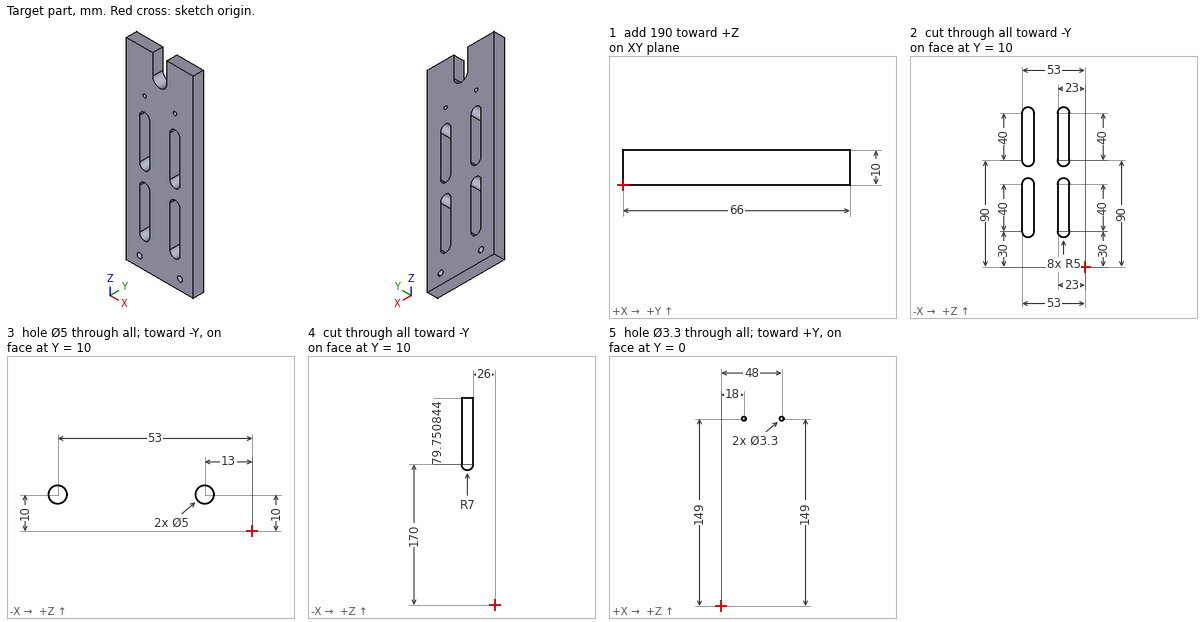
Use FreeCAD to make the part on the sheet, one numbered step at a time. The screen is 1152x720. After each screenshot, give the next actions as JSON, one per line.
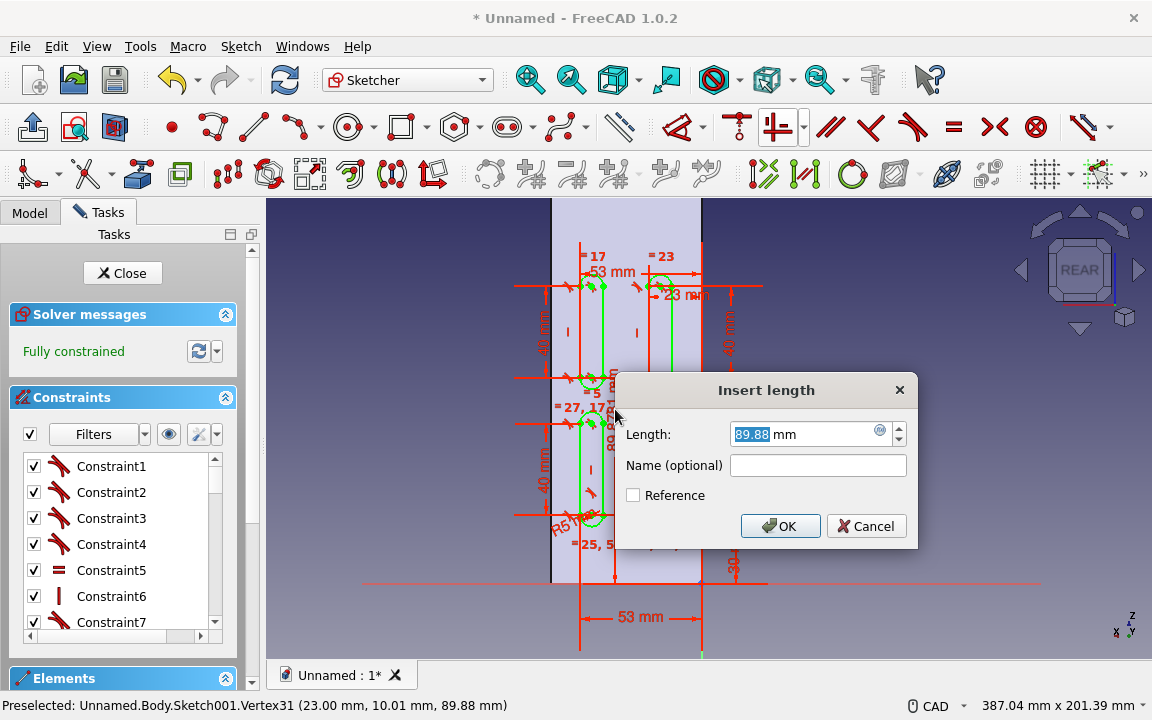
{"action": "type", "text": "90"}
{"action": "key", "text": "Return"}
{"action": "key", "text": "Escape"}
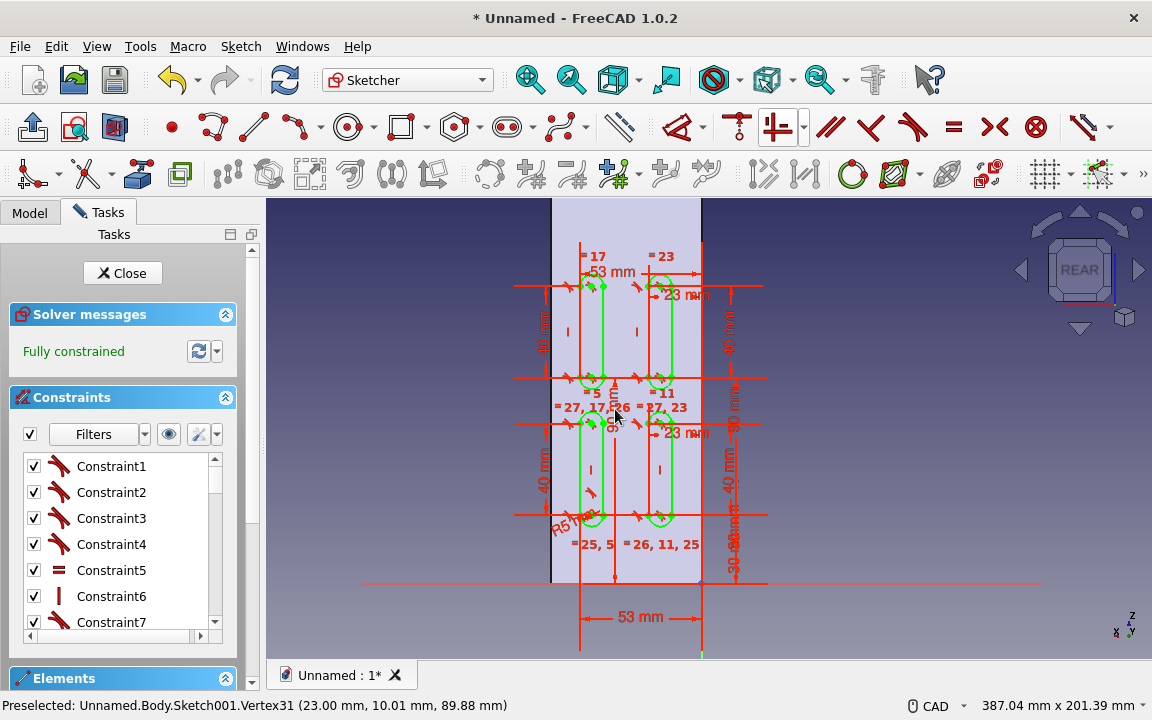
{"action": "left_click", "coordinate": [123, 273]}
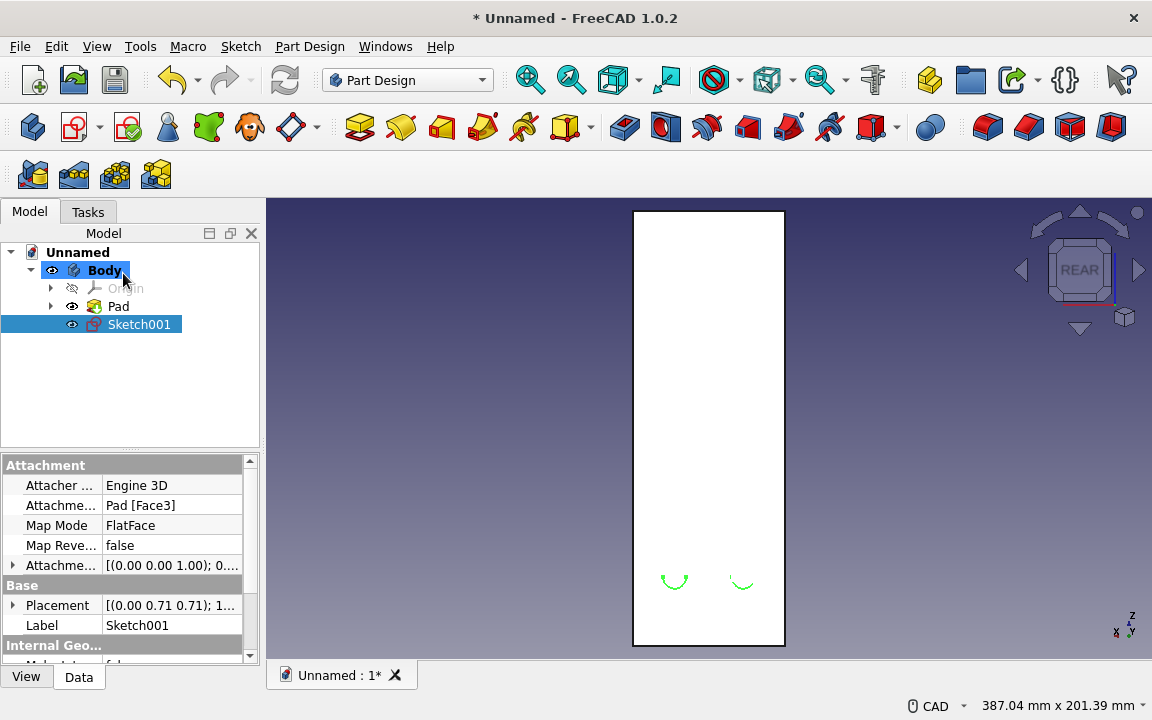
{"action": "left_click", "coordinate": [625, 128]}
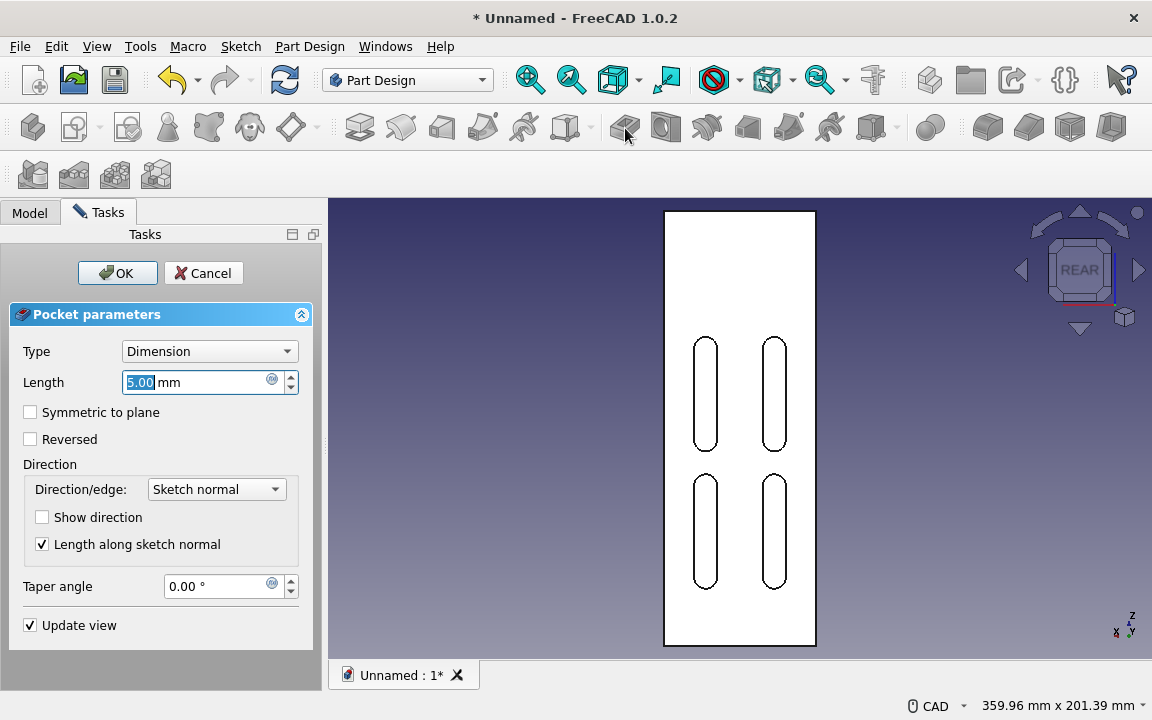
{"action": "left_click", "coordinate": [210, 352]}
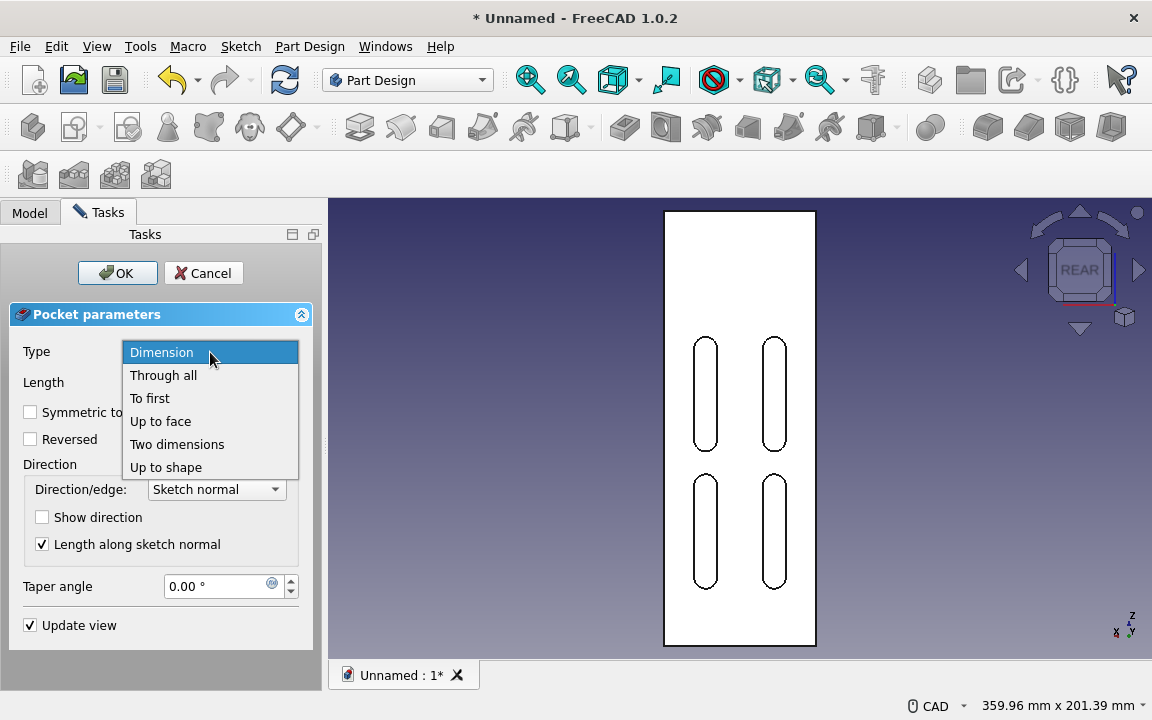
{"action": "left_click", "coordinate": [208, 376]}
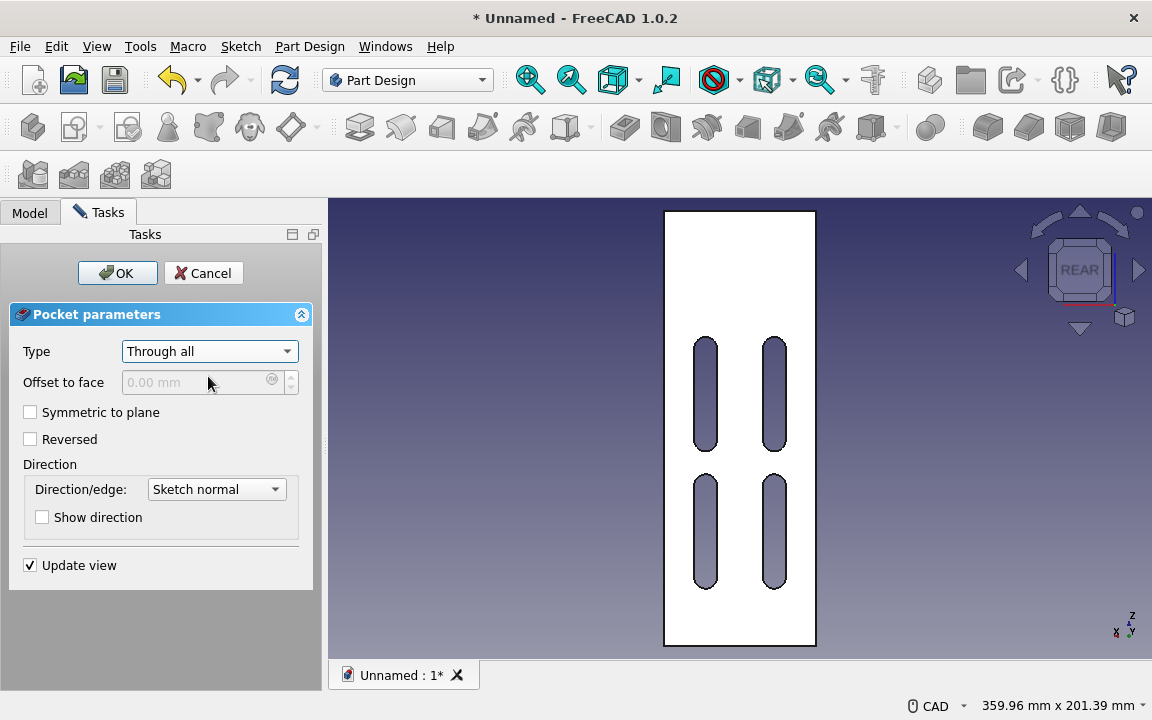
{"action": "left_click", "coordinate": [118, 273]}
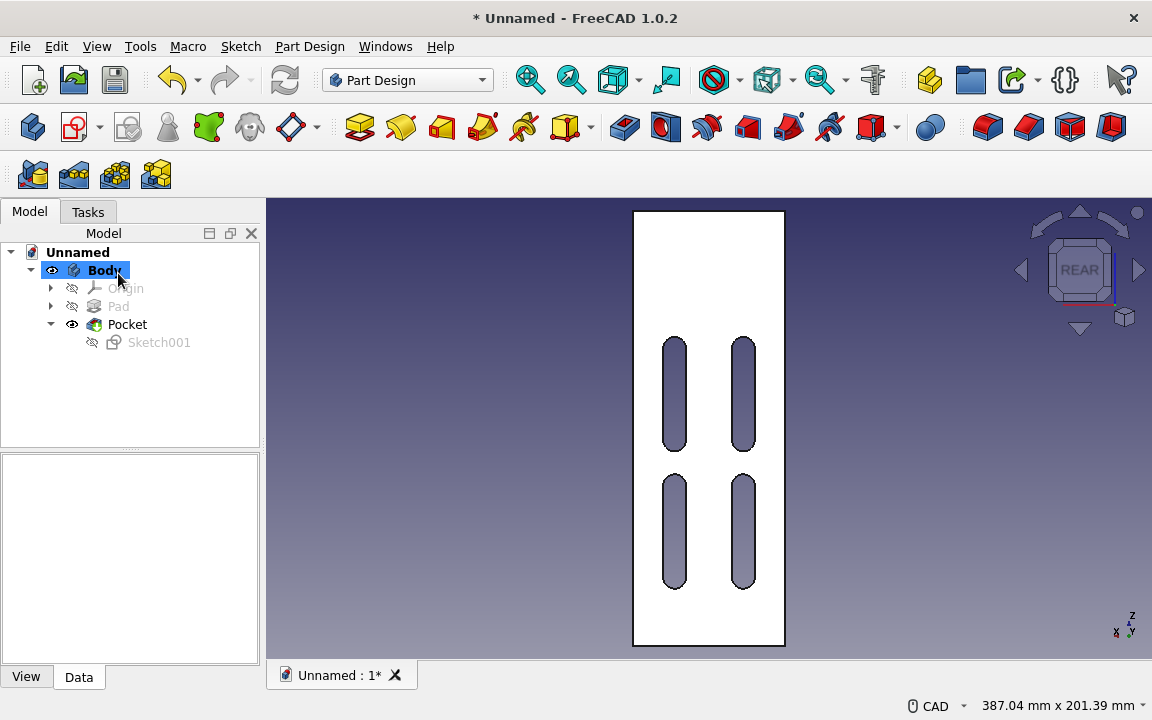
{"action": "left_click", "coordinate": [709, 303]}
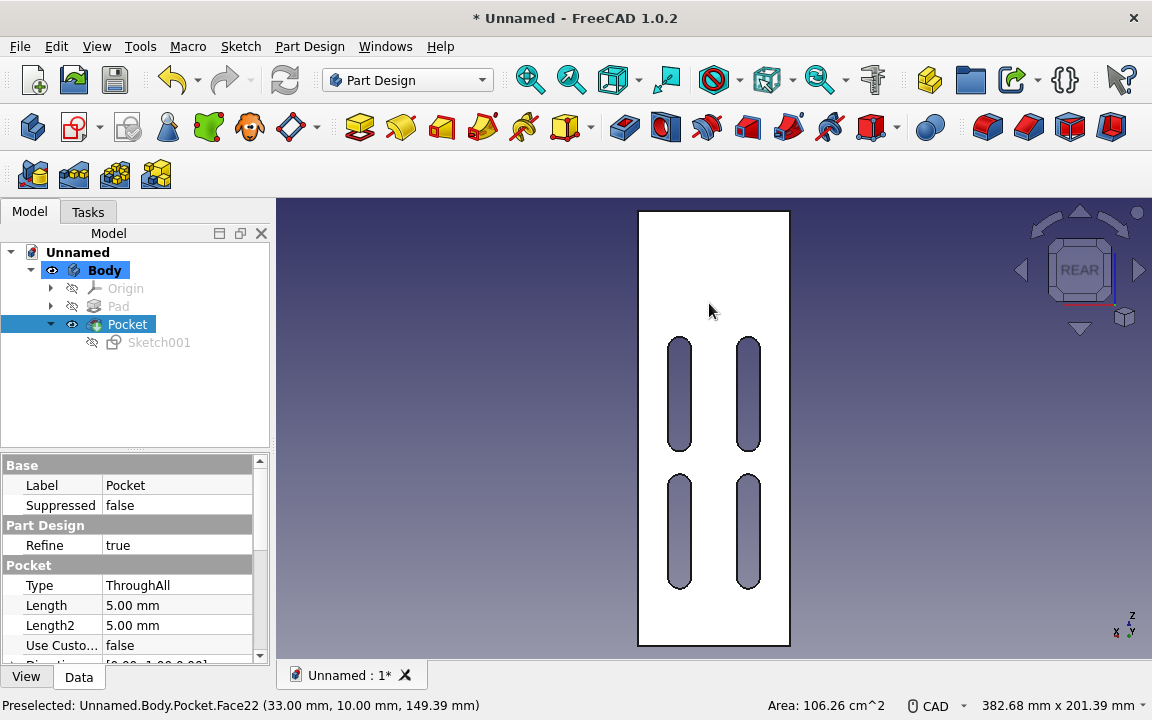
{"action": "left_click", "coordinate": [74, 128]}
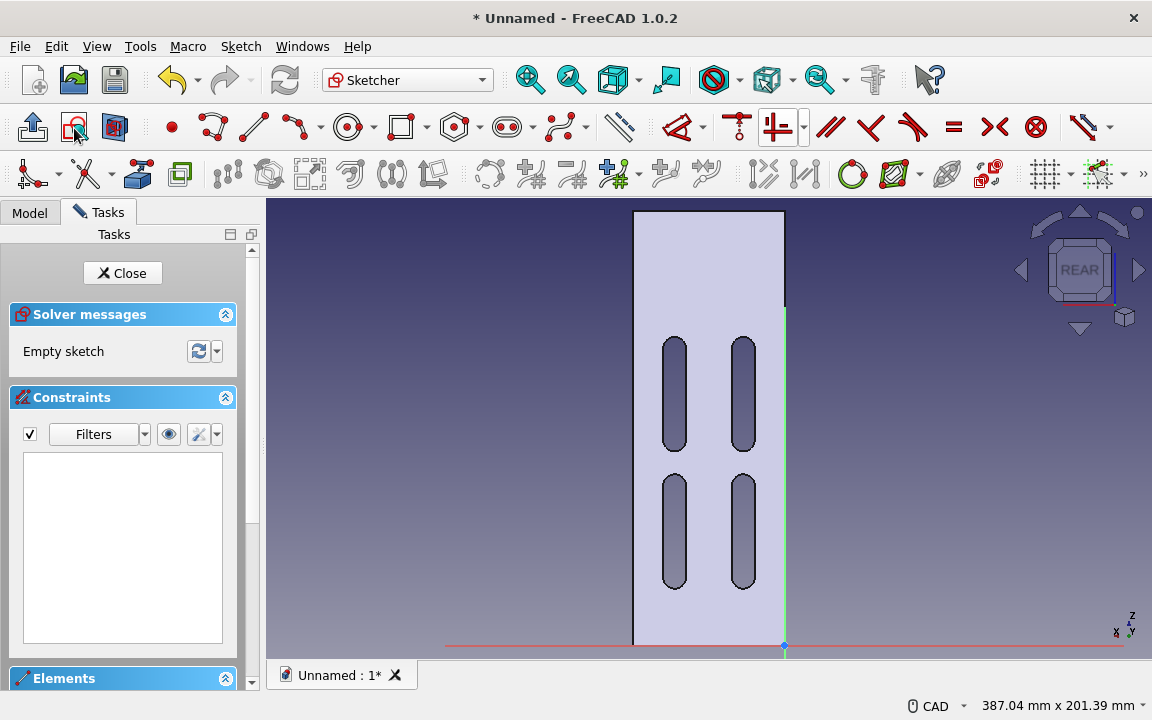
{"action": "scroll", "coordinate": [640, 428], "scroll_direction": "down", "scroll_amount": 5}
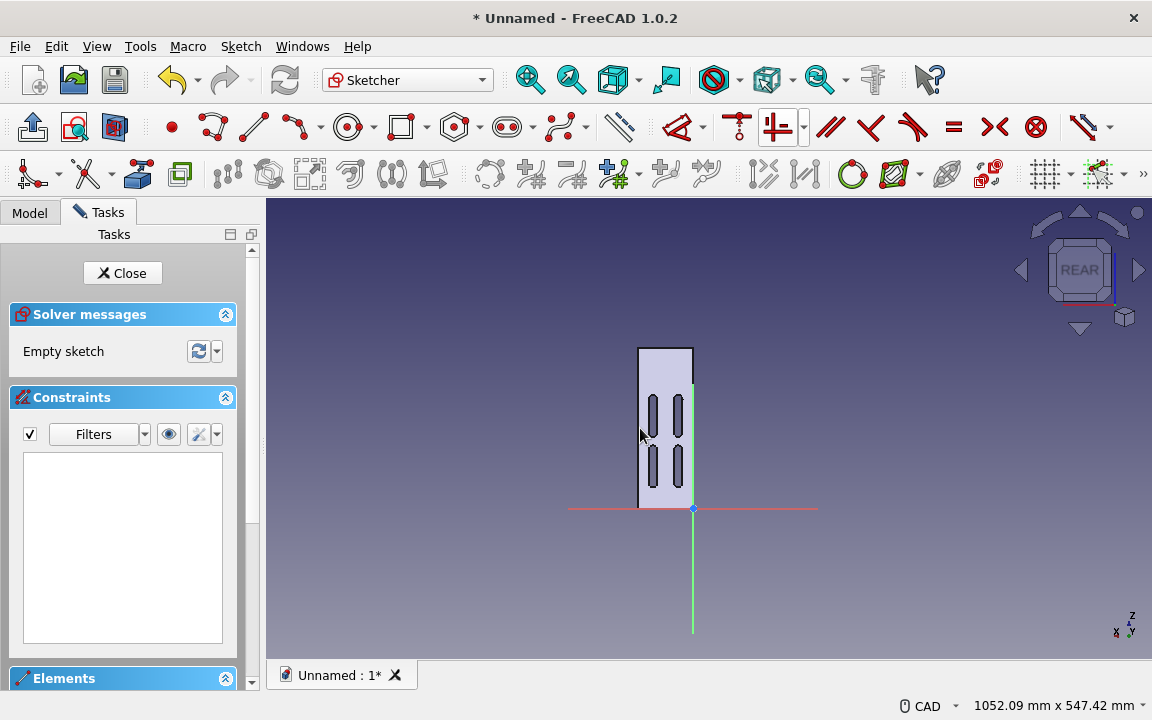
{"action": "scroll", "coordinate": [673, 511], "scroll_direction": "up", "scroll_amount": 12}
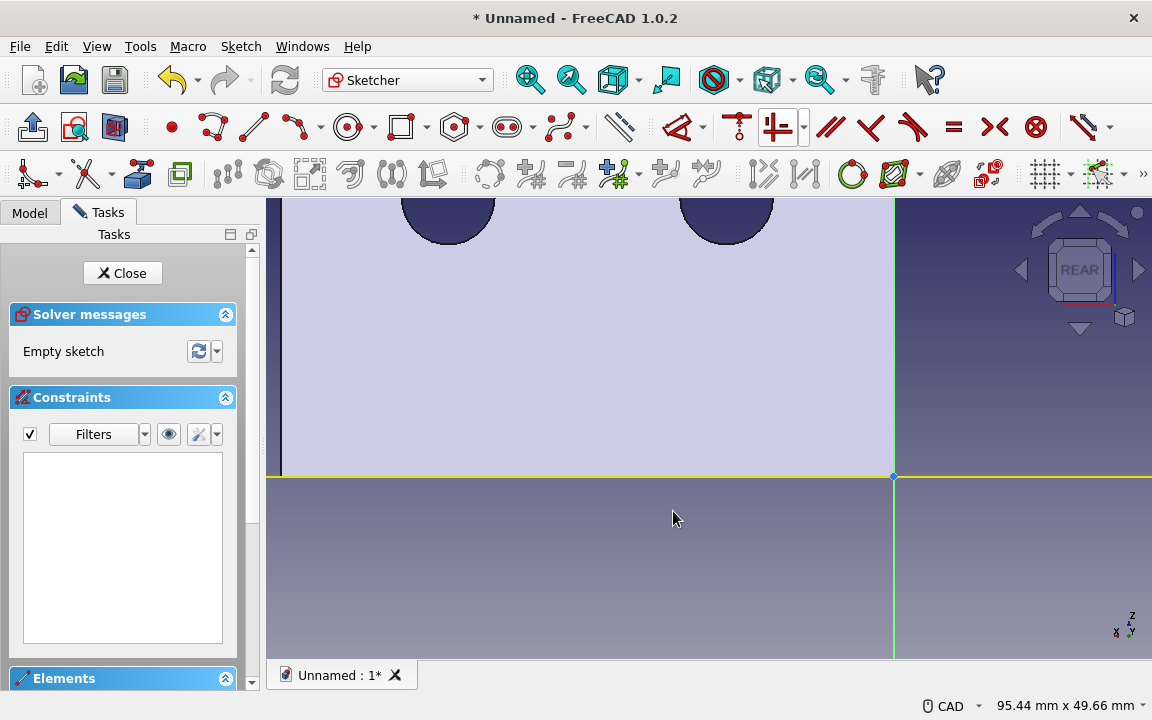
{"action": "left_click", "coordinate": [348, 128]}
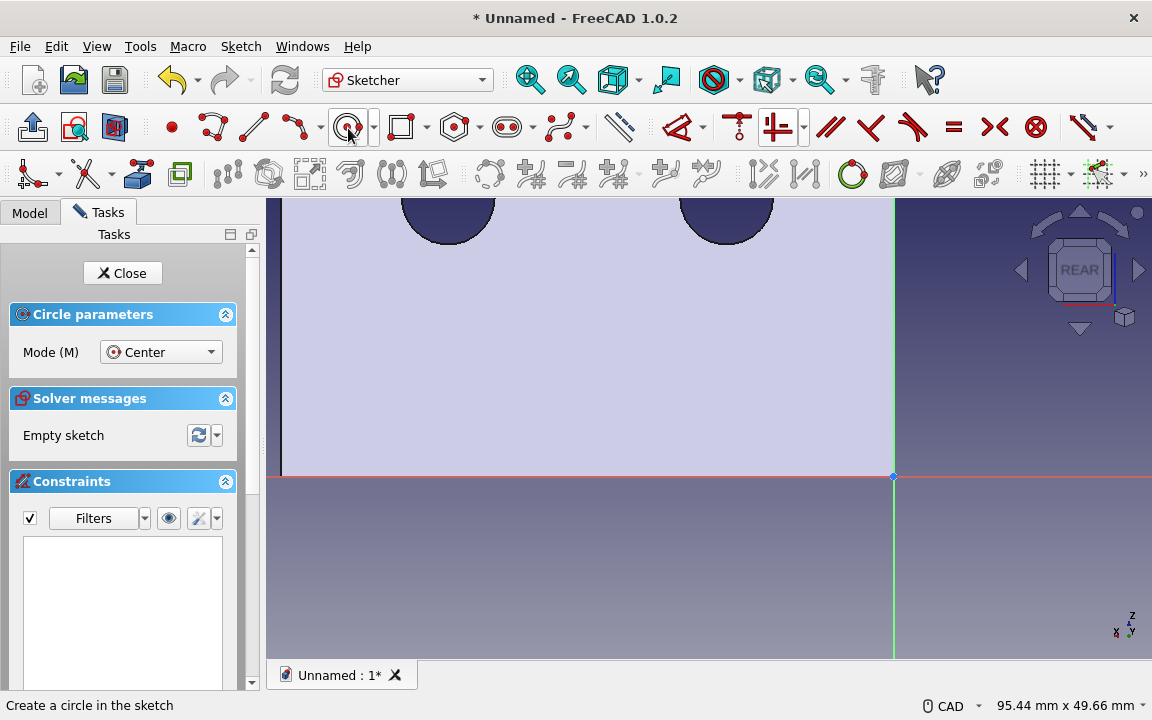
{"action": "left_click", "coordinate": [773, 384]}
{"action": "mouse_move", "coordinate": [789, 367]}